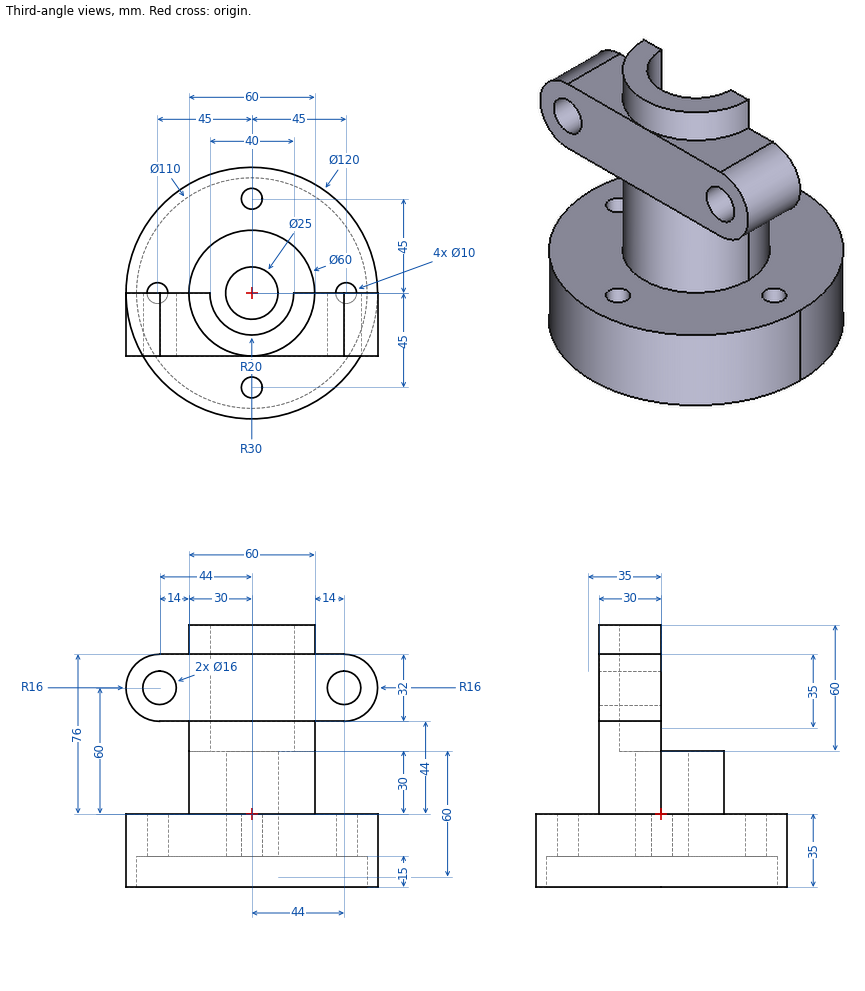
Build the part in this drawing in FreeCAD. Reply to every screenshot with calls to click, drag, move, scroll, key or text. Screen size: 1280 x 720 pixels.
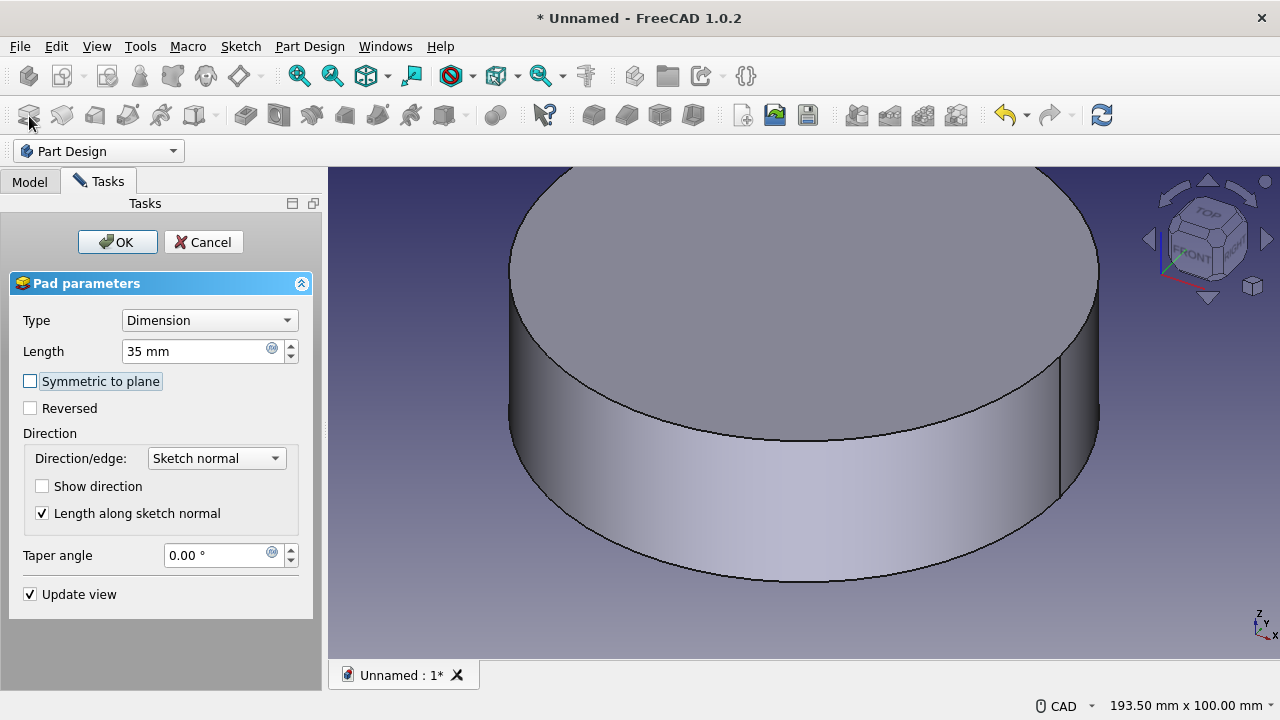
click(31, 408)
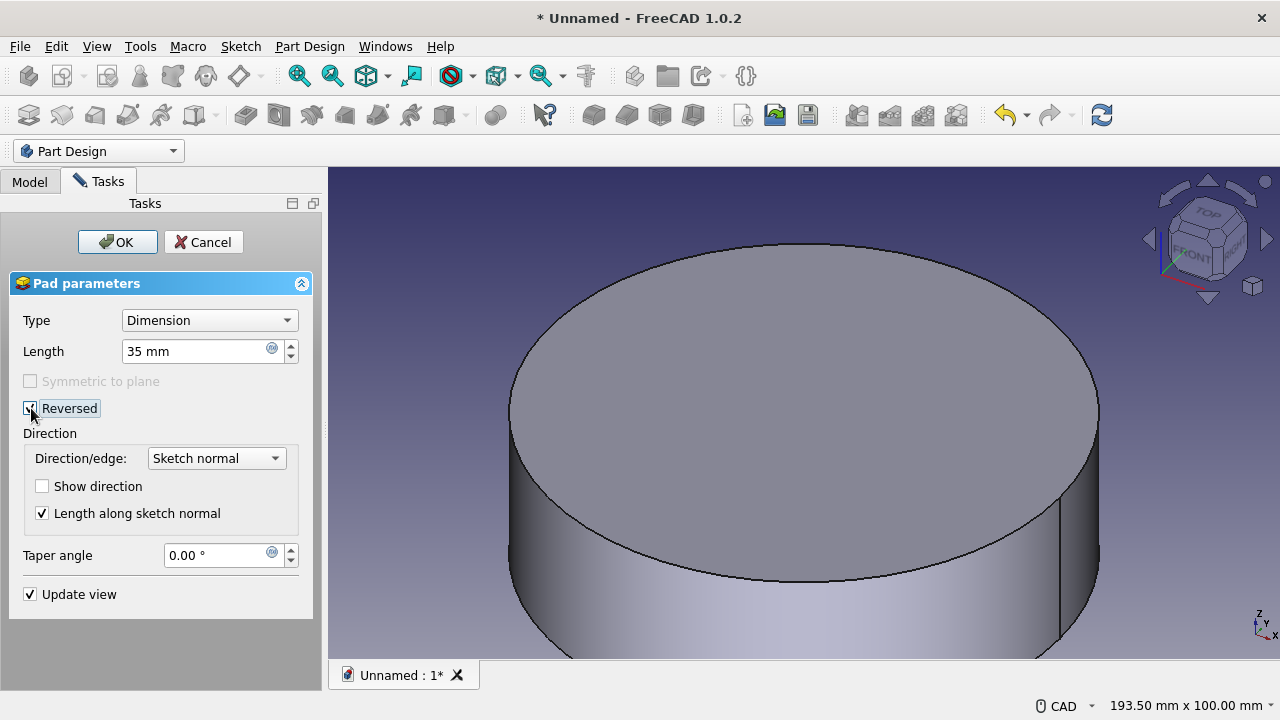
click(118, 242)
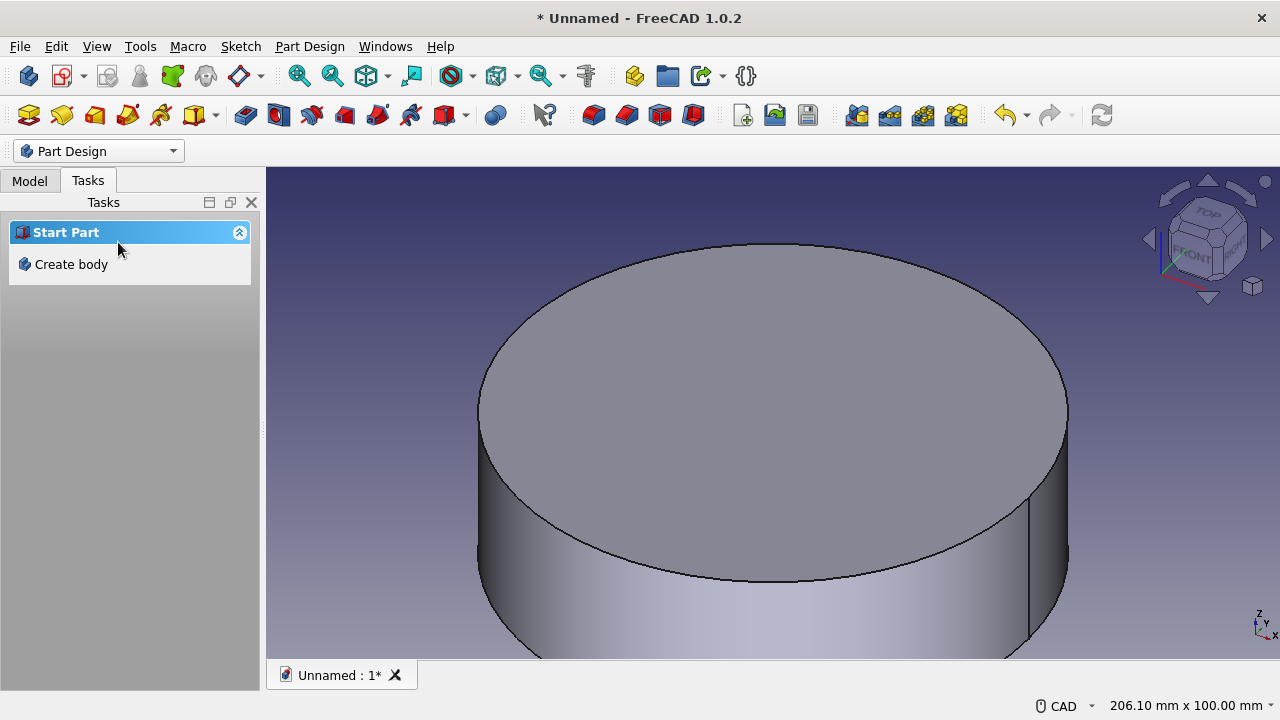
click(300, 76)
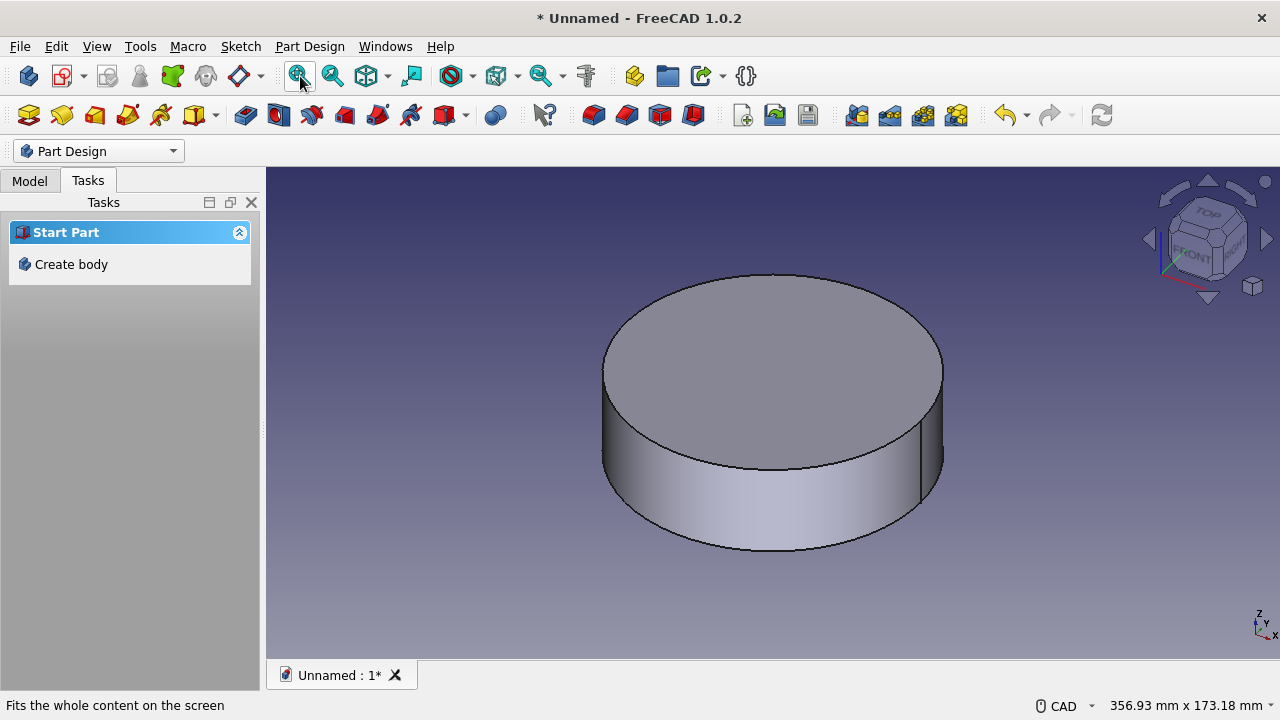
click(62, 76)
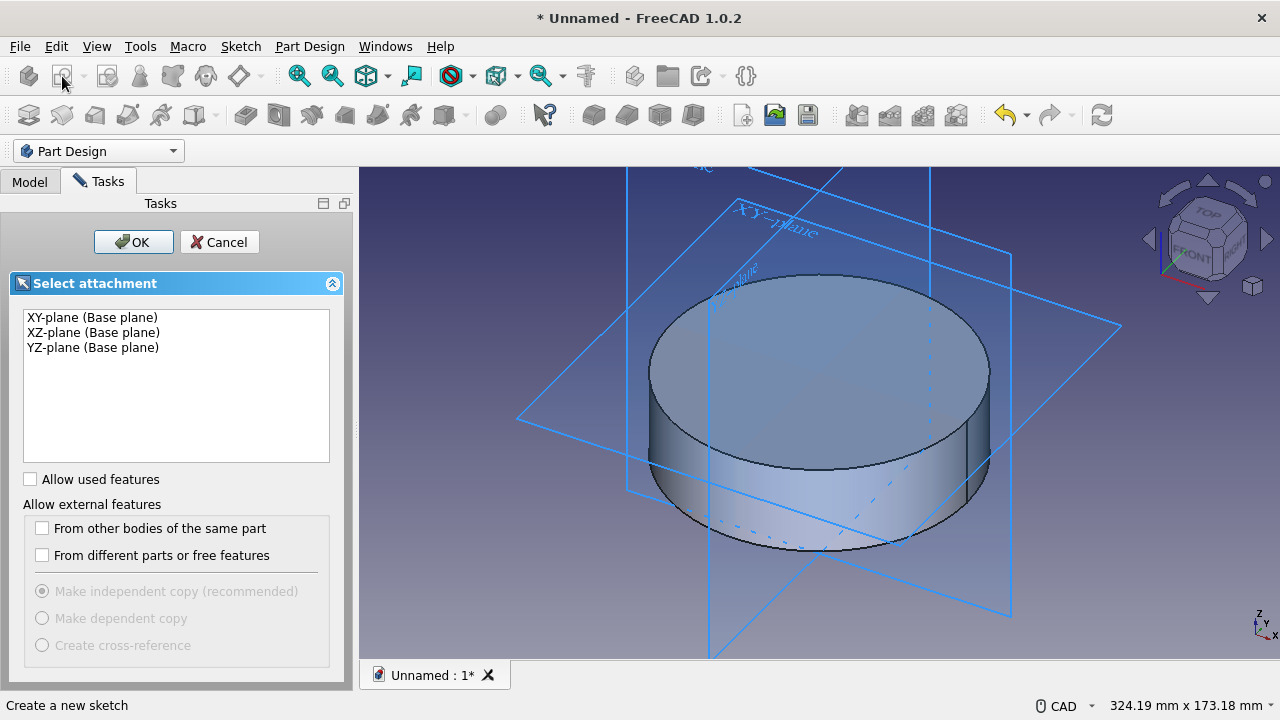
click(84, 318)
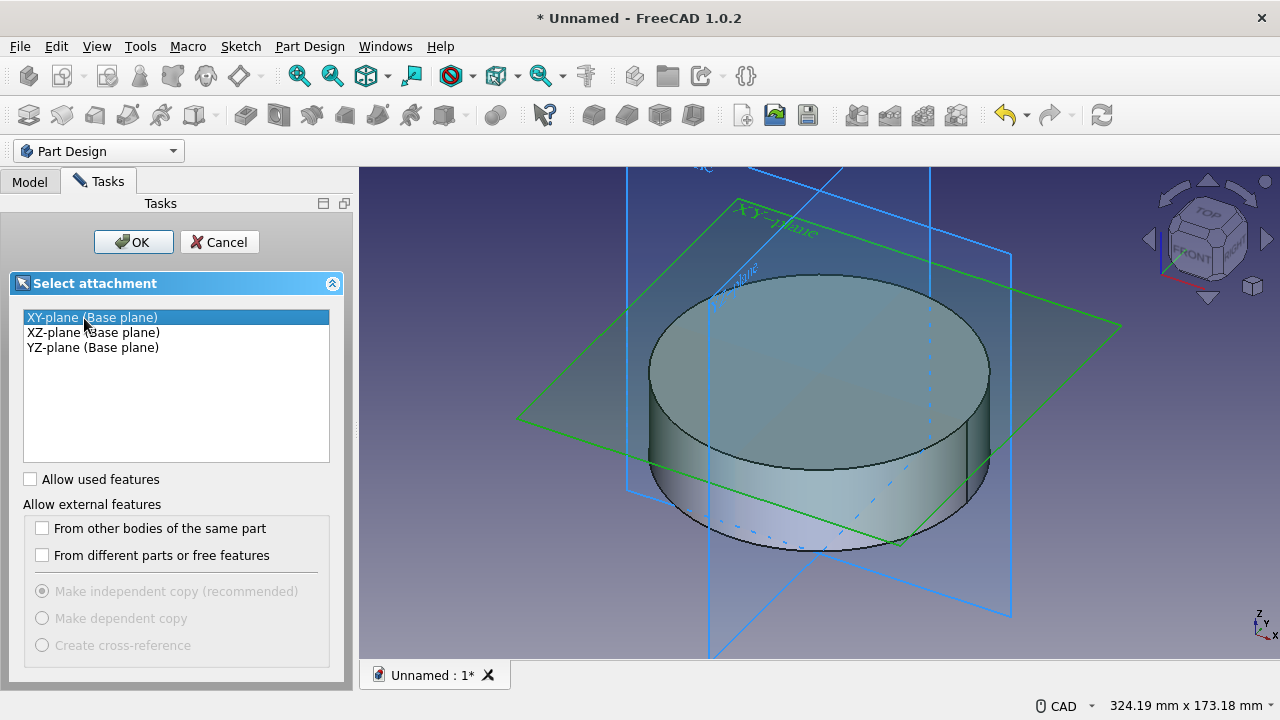
click(134, 242)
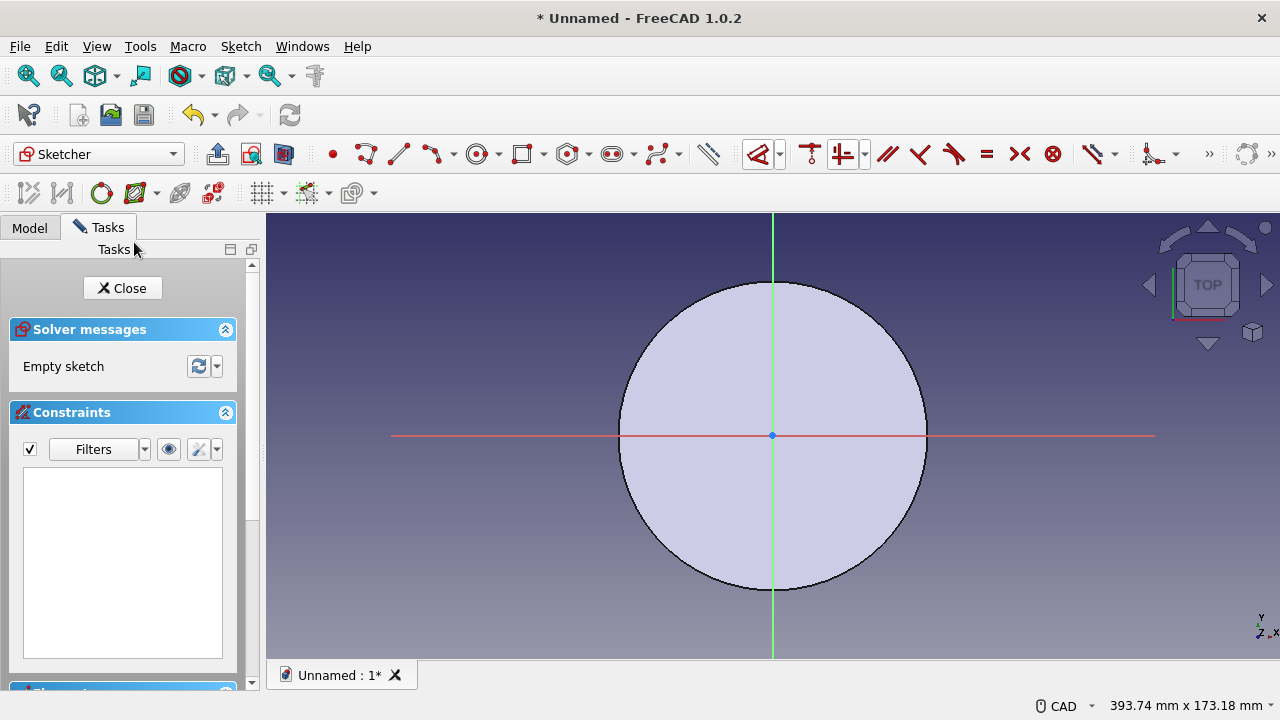
scroll(856, 436, up, 3)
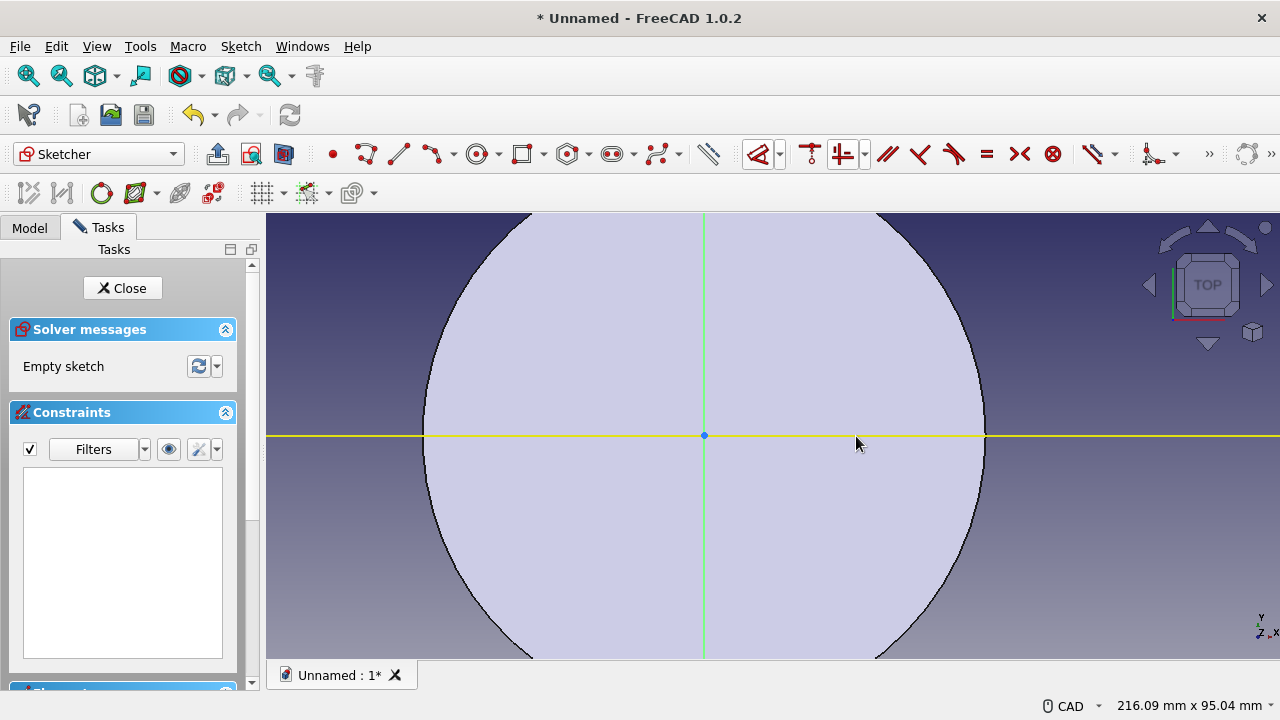
click(476, 154)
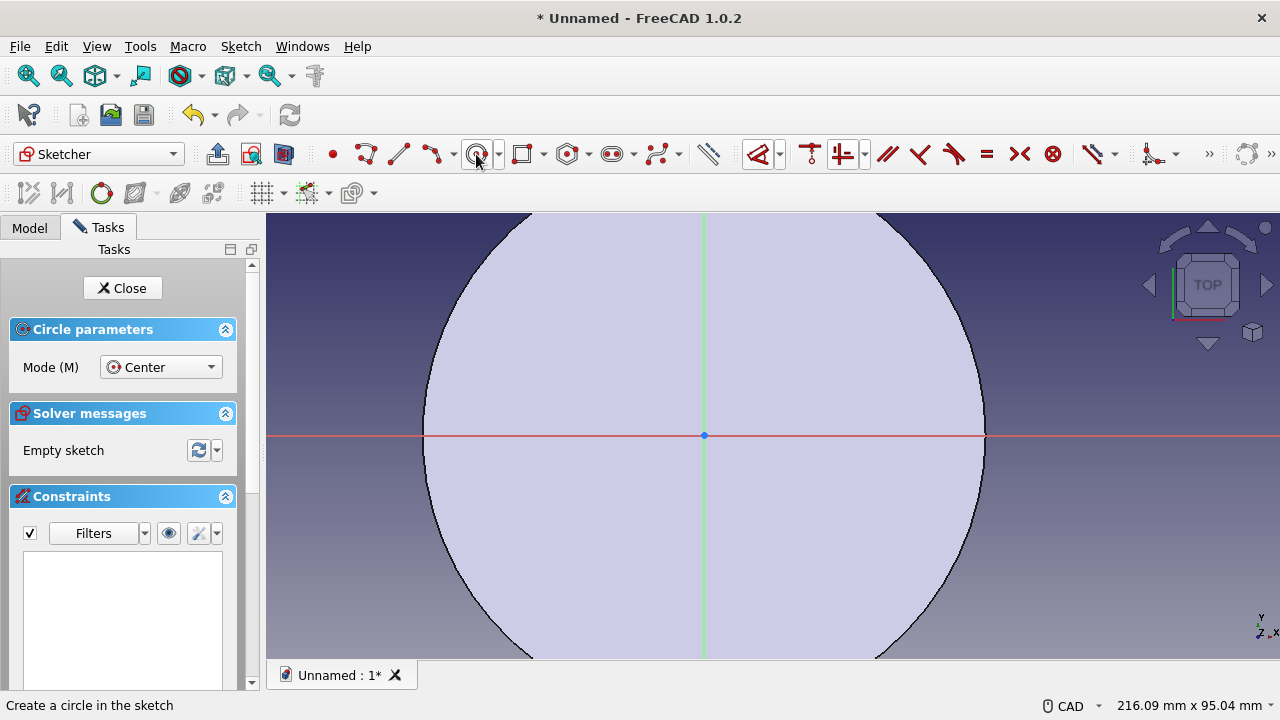
click(704, 436)
move(804, 336)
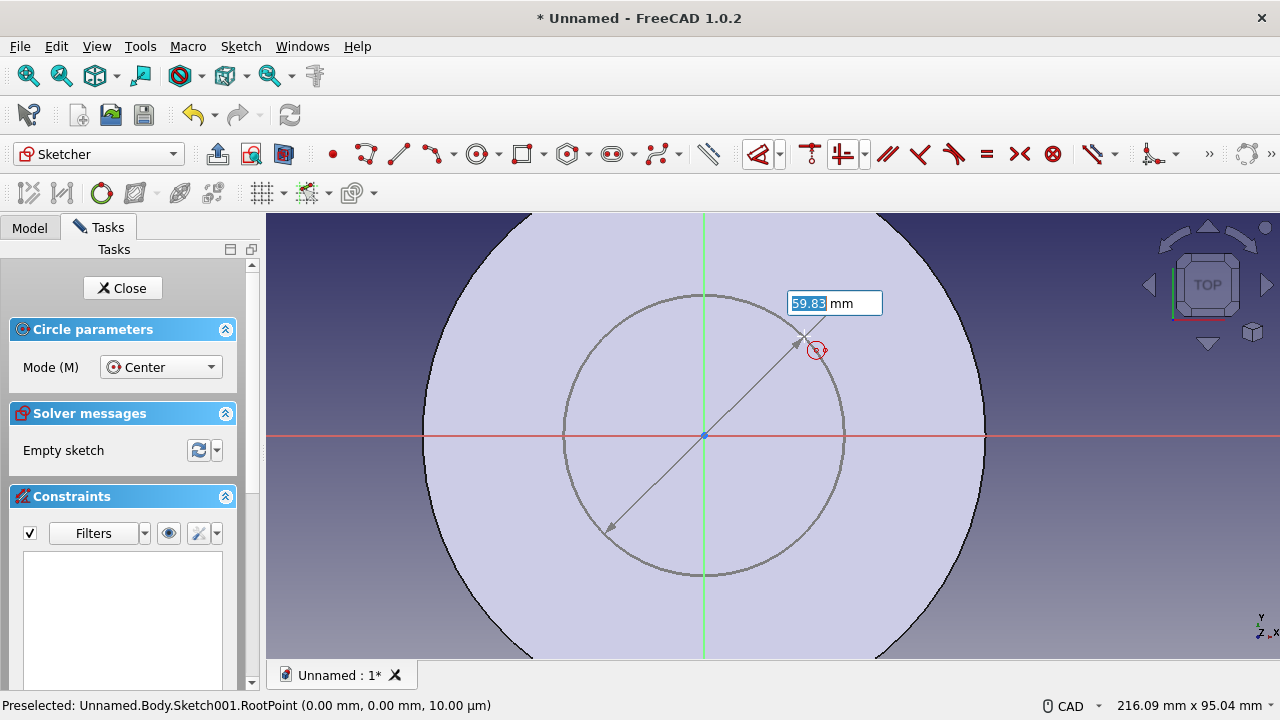
text(60)
key(Return)
key(Escape)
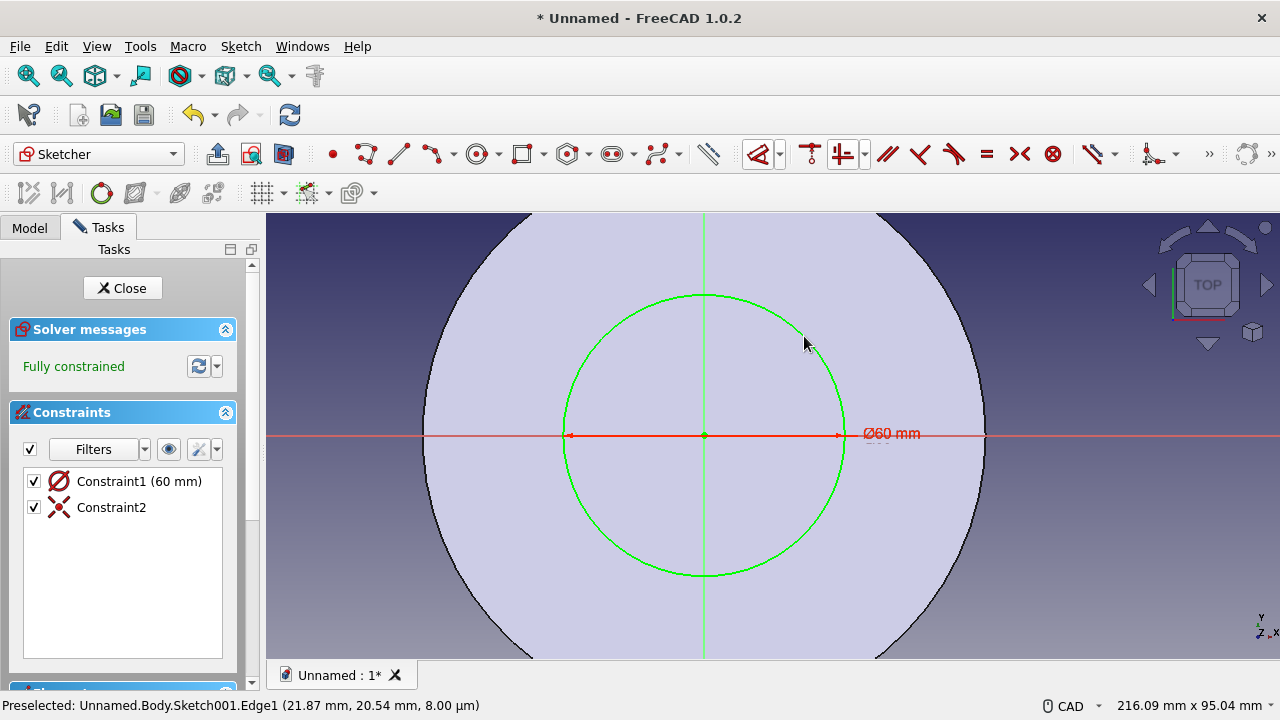
click(123, 288)